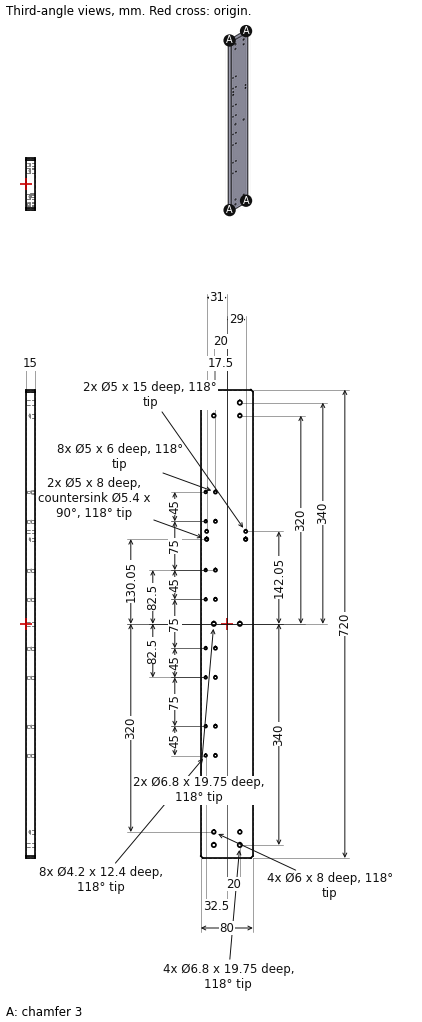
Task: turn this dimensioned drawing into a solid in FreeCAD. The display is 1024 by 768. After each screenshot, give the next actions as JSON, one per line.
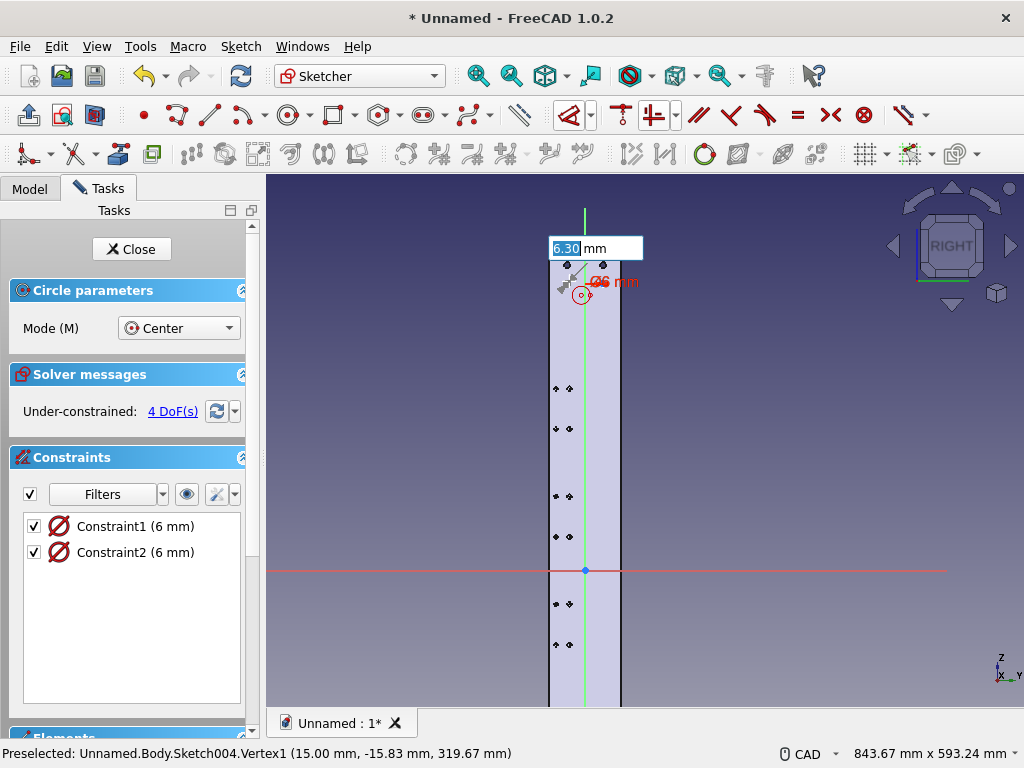
{"action": "type", "text": "6"}
{"action": "key", "text": "Return"}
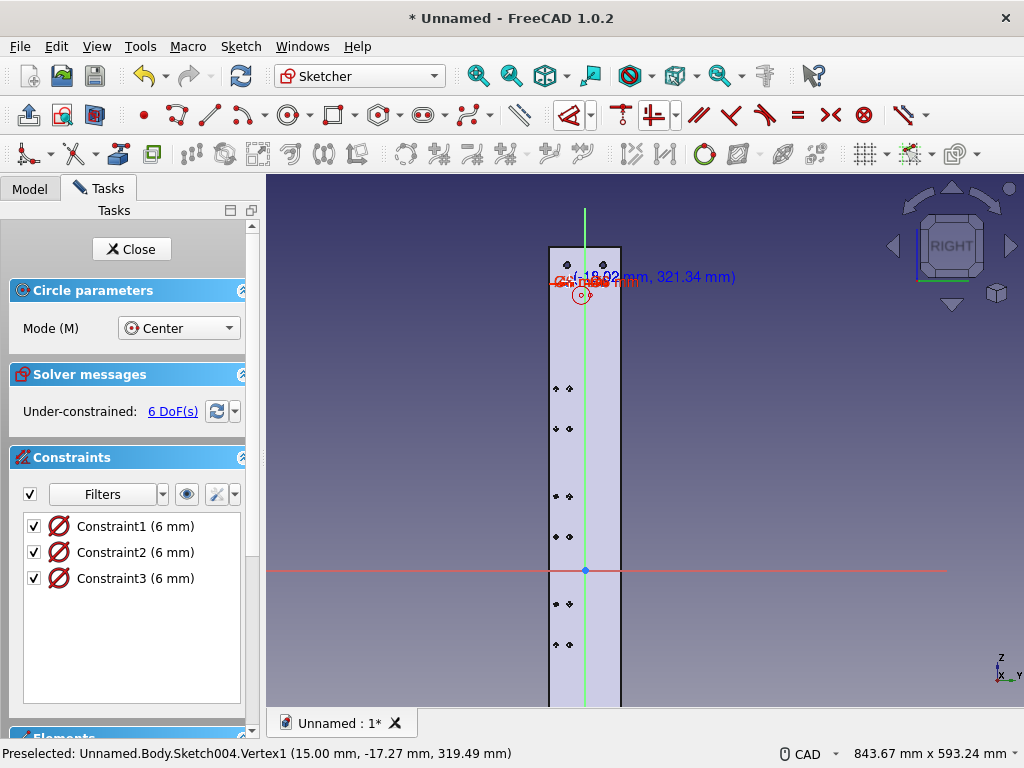
{"action": "scroll", "coordinate": [566, 282], "scroll_direction": "down", "scroll_amount": 3}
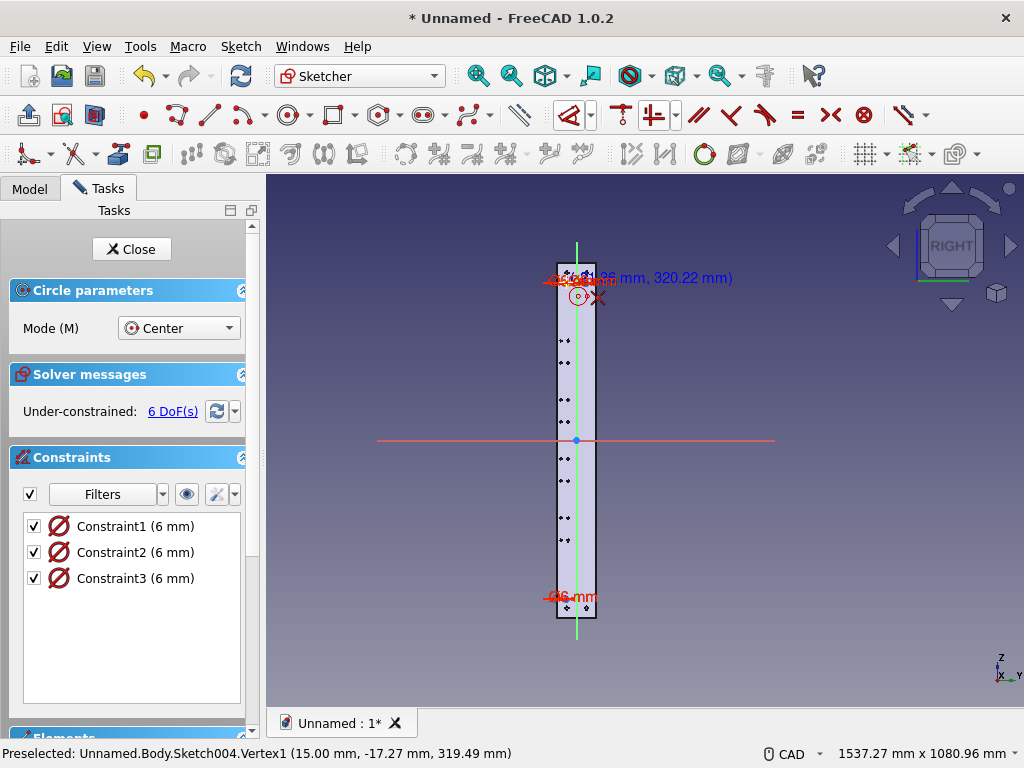
{"action": "scroll", "coordinate": [587, 598], "scroll_direction": "up", "scroll_amount": 14}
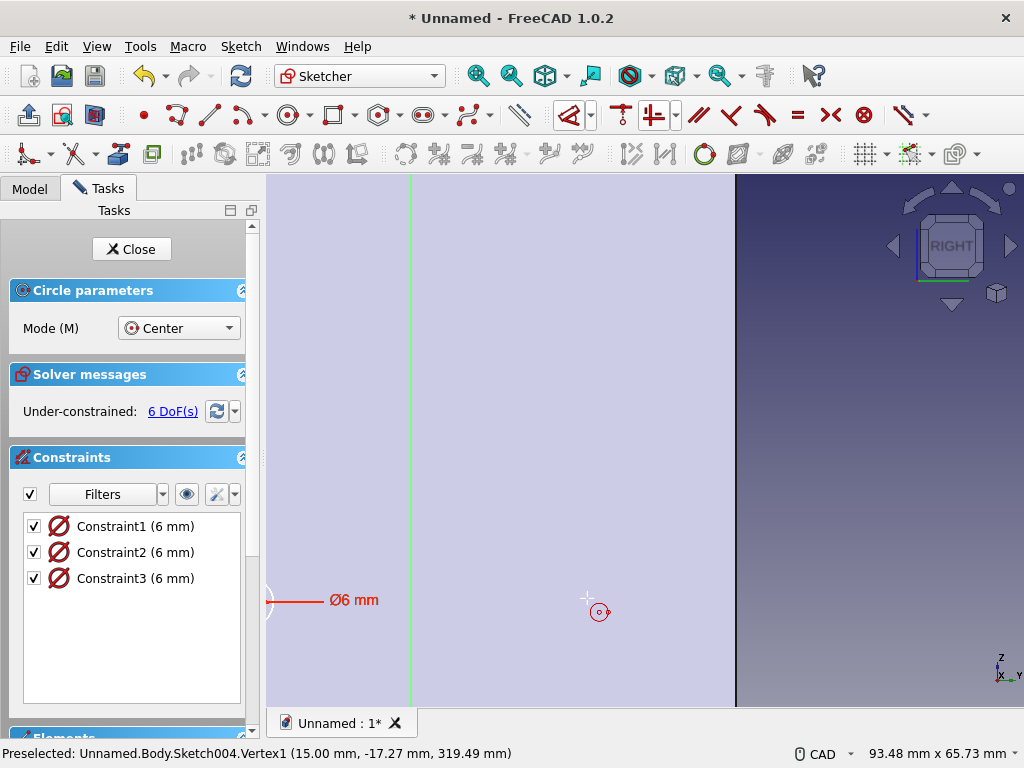
{"action": "scroll", "coordinate": [587, 599], "scroll_direction": "down", "scroll_amount": 14}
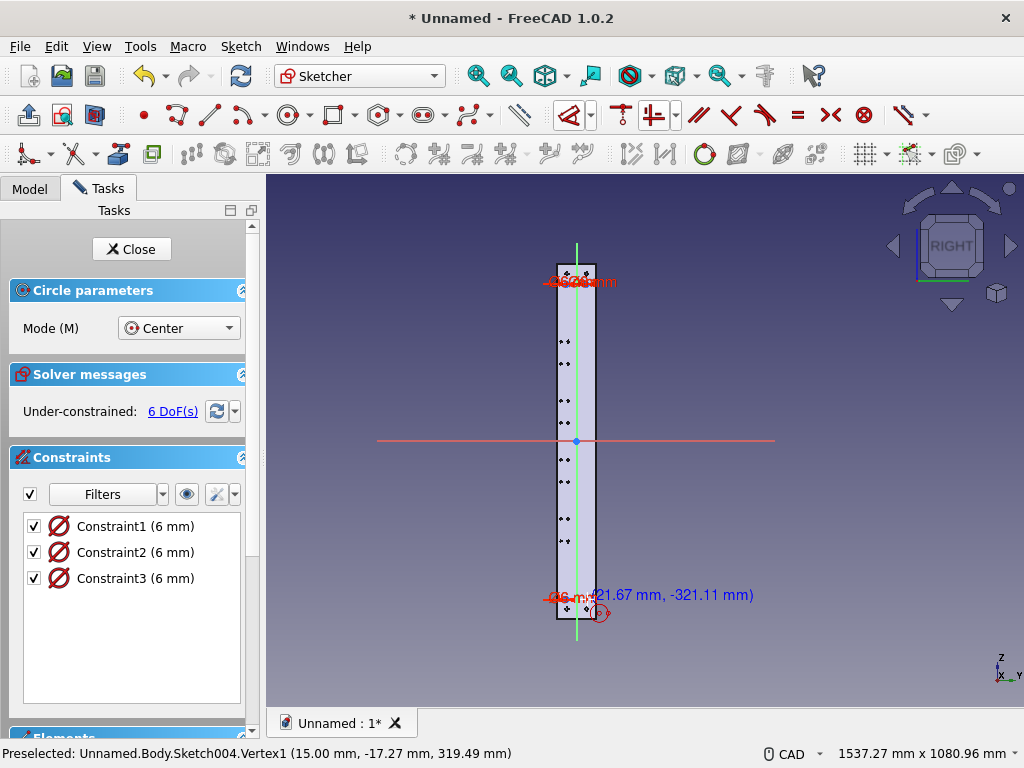
{"action": "scroll", "coordinate": [587, 599], "scroll_direction": "up", "scroll_amount": 3}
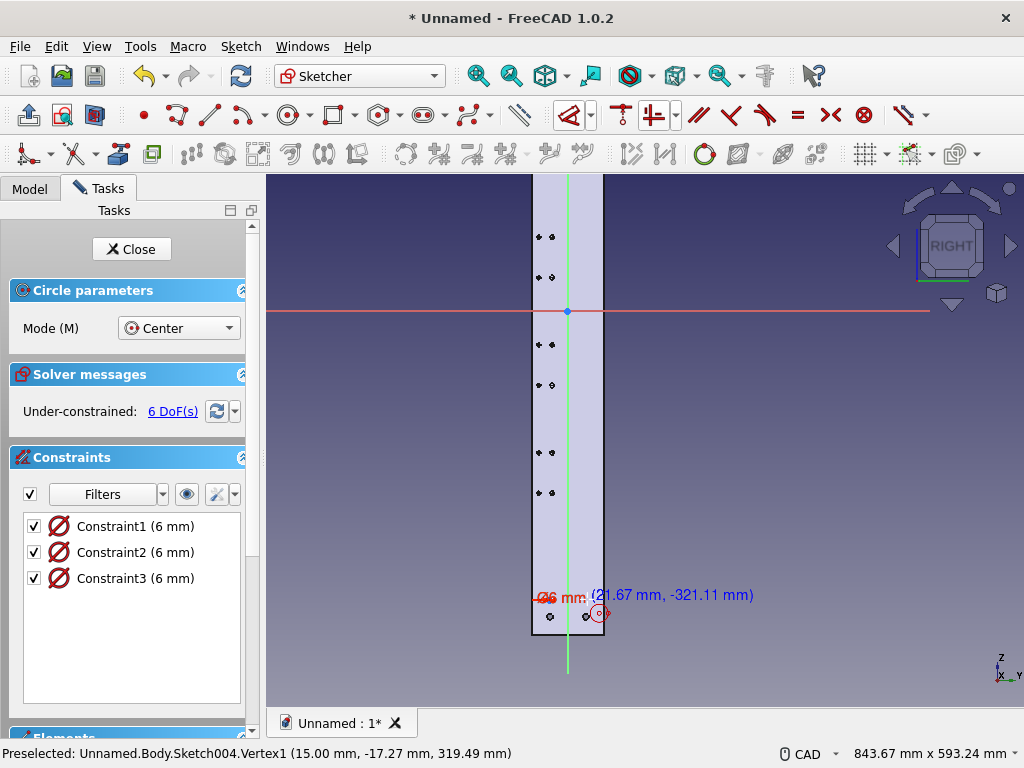
{"action": "left_click", "coordinate": [586, 599]}
{"action": "mouse_move", "coordinate": [588, 597]}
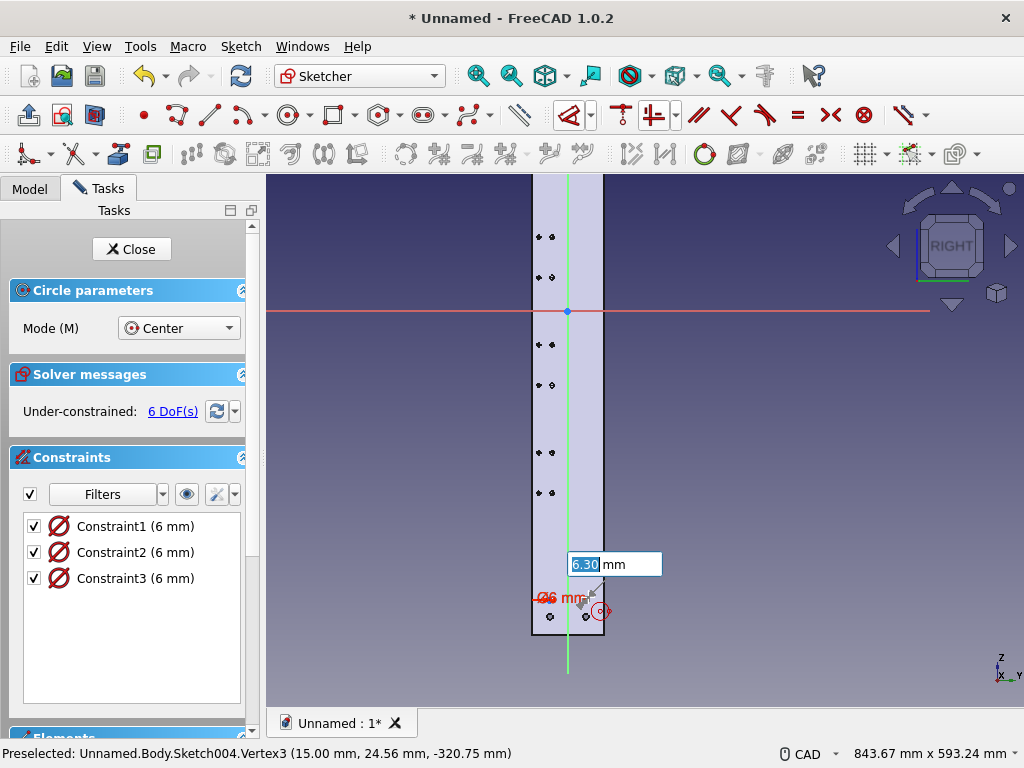
{"action": "type", "text": "6"}
{"action": "key", "text": "Return"}
{"action": "key", "text": "Escape"}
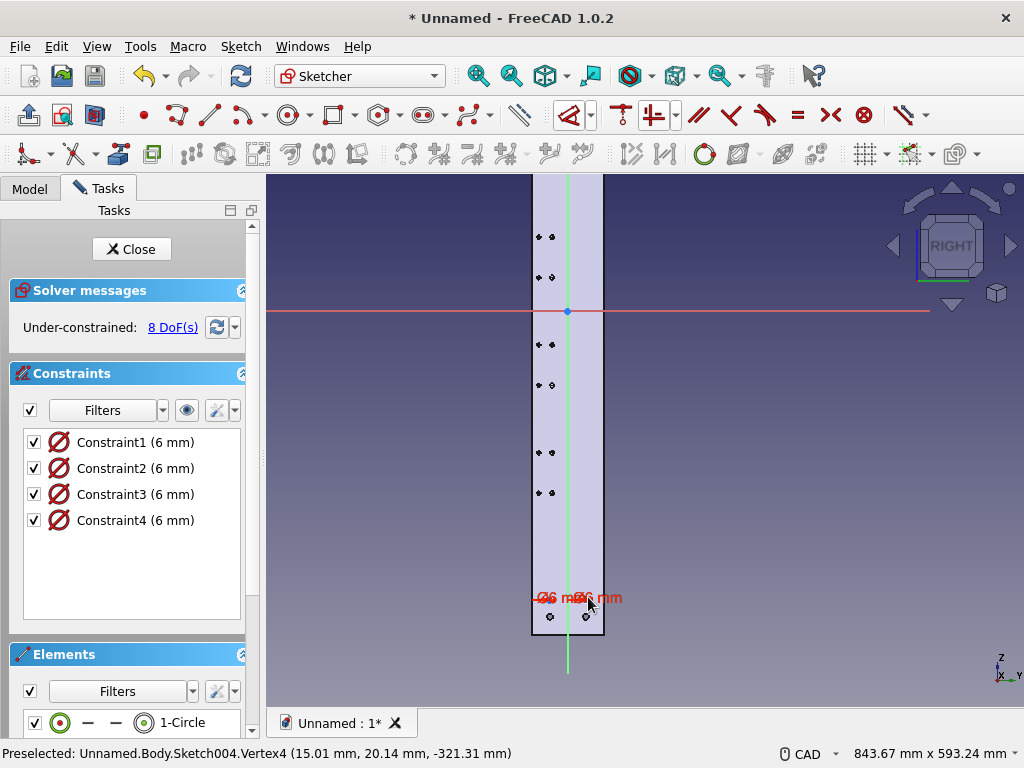
{"action": "left_click", "coordinate": [550, 600]}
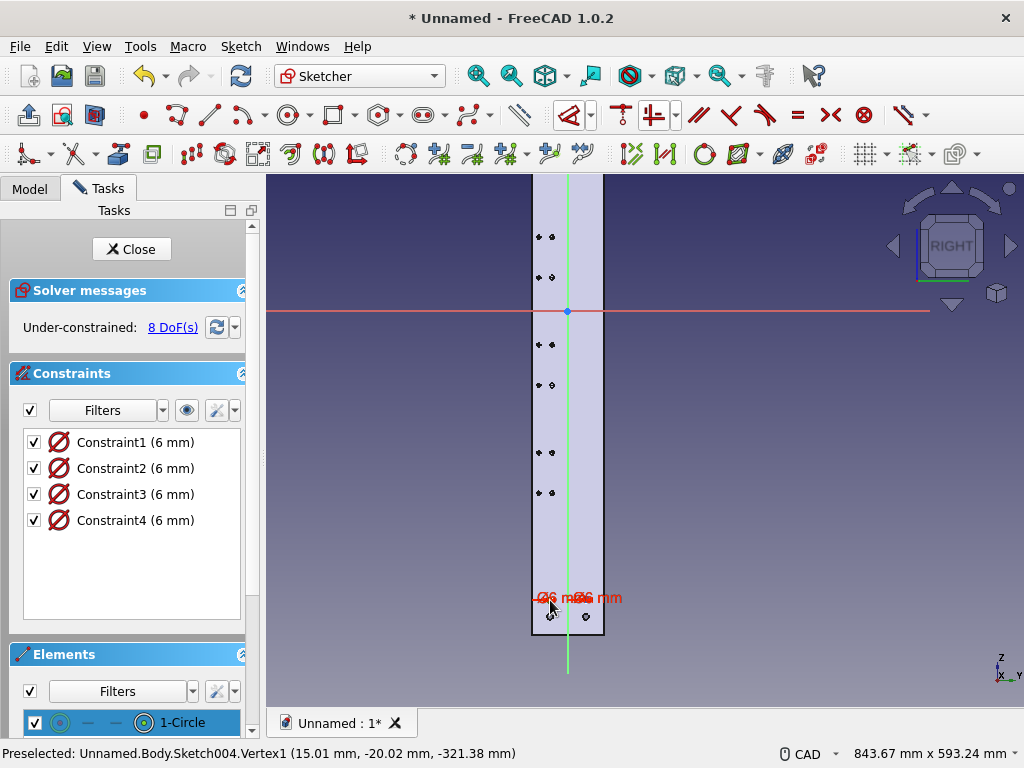
{"action": "scroll", "coordinate": [587, 598], "scroll_direction": "down", "scroll_amount": 3}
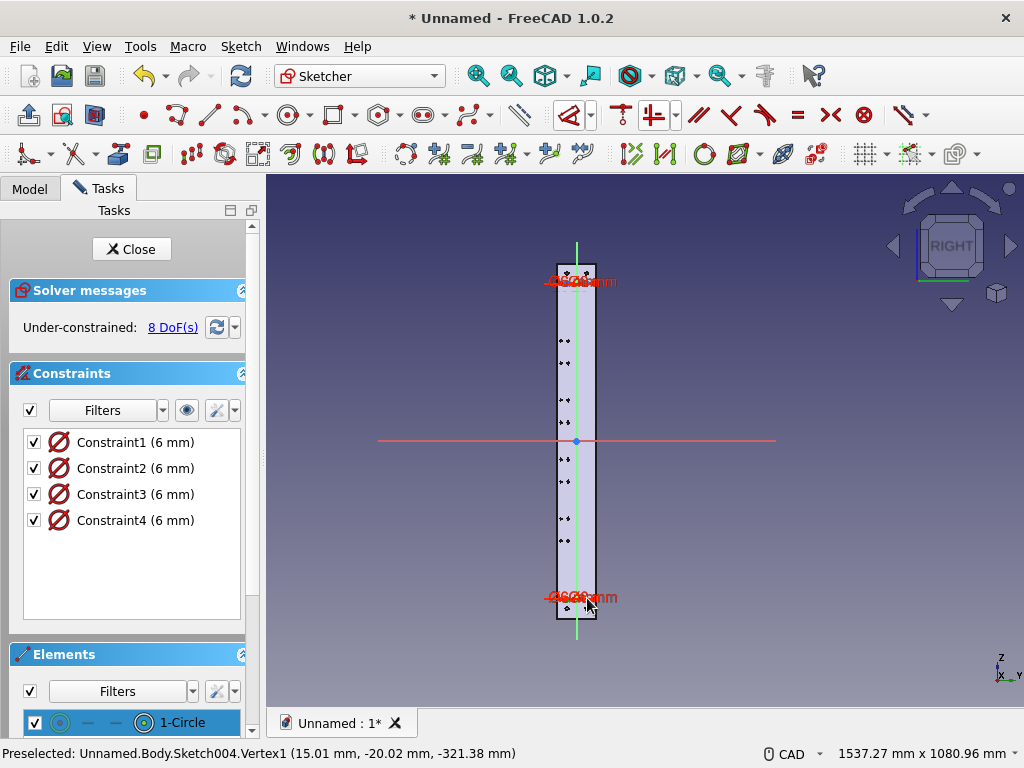
{"action": "left_click", "coordinate": [567, 284]}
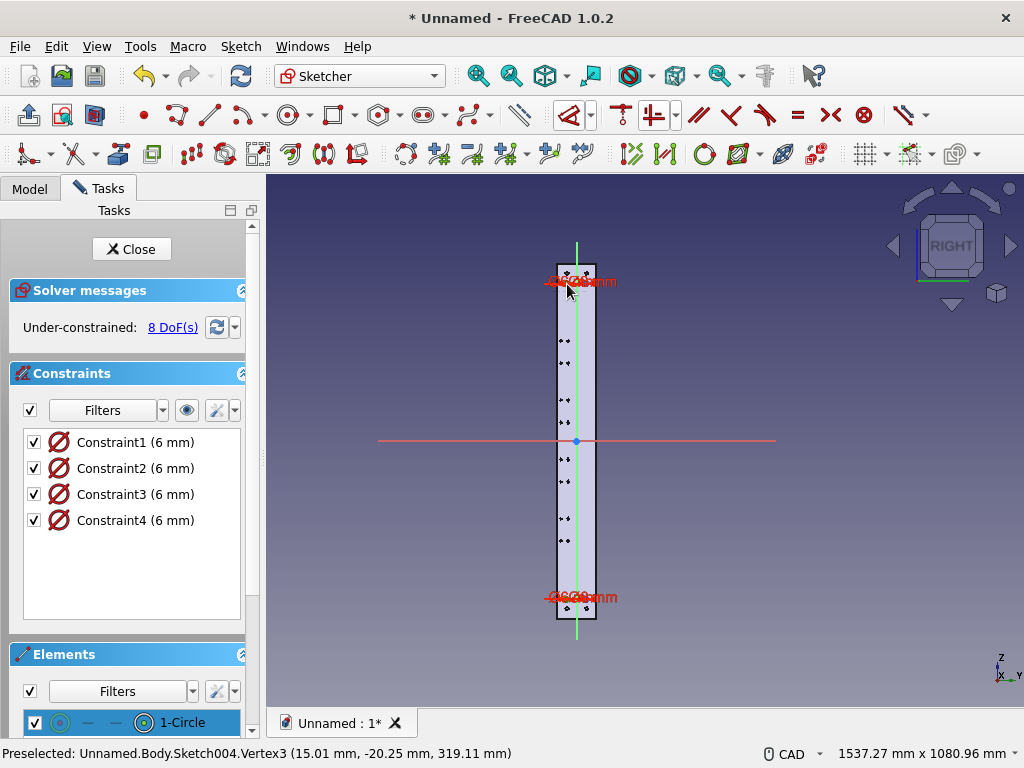
{"action": "left_click", "coordinate": [676, 116]}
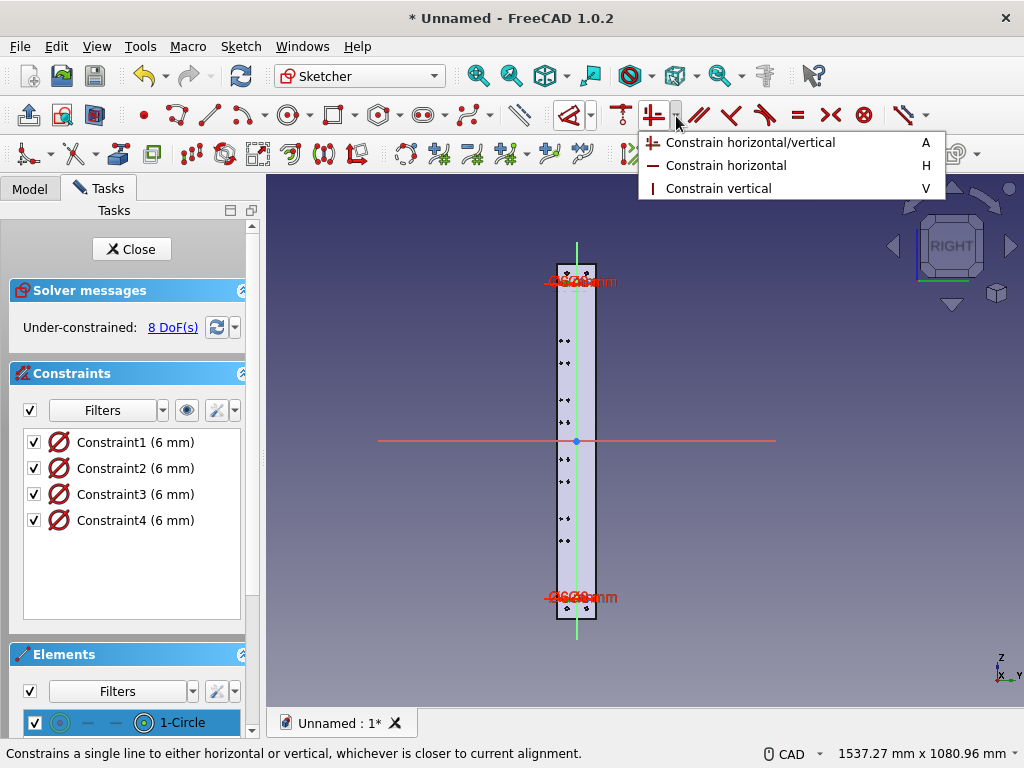
{"action": "left_click", "coordinate": [792, 188]}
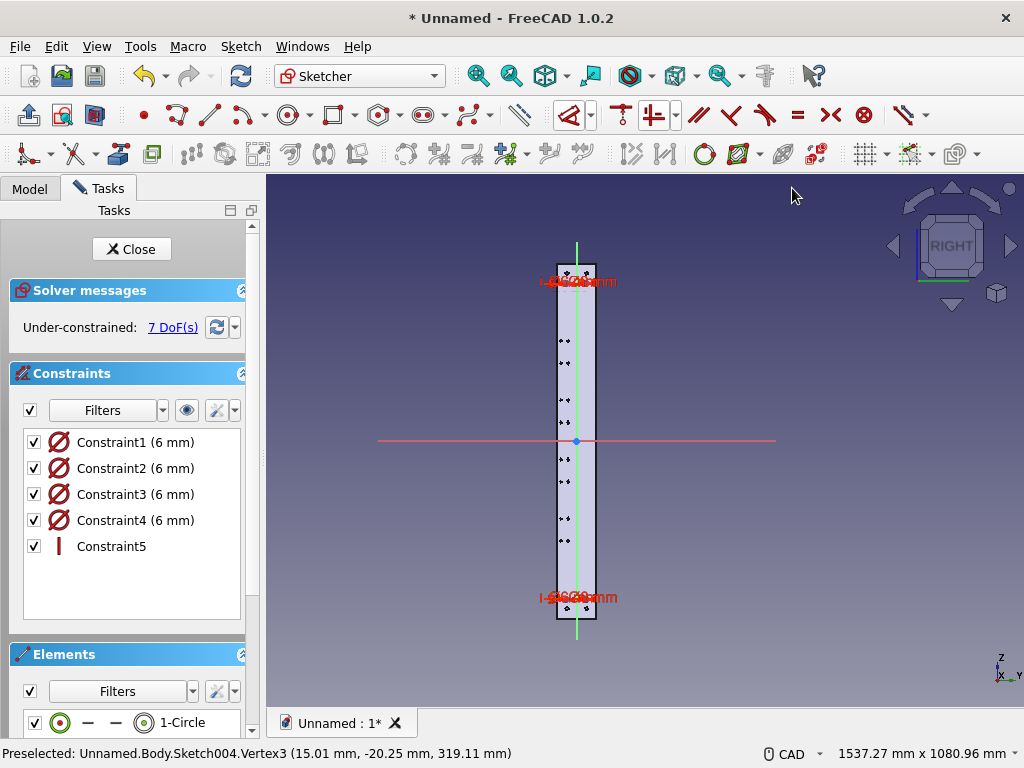
{"action": "left_click", "coordinate": [586, 284]}